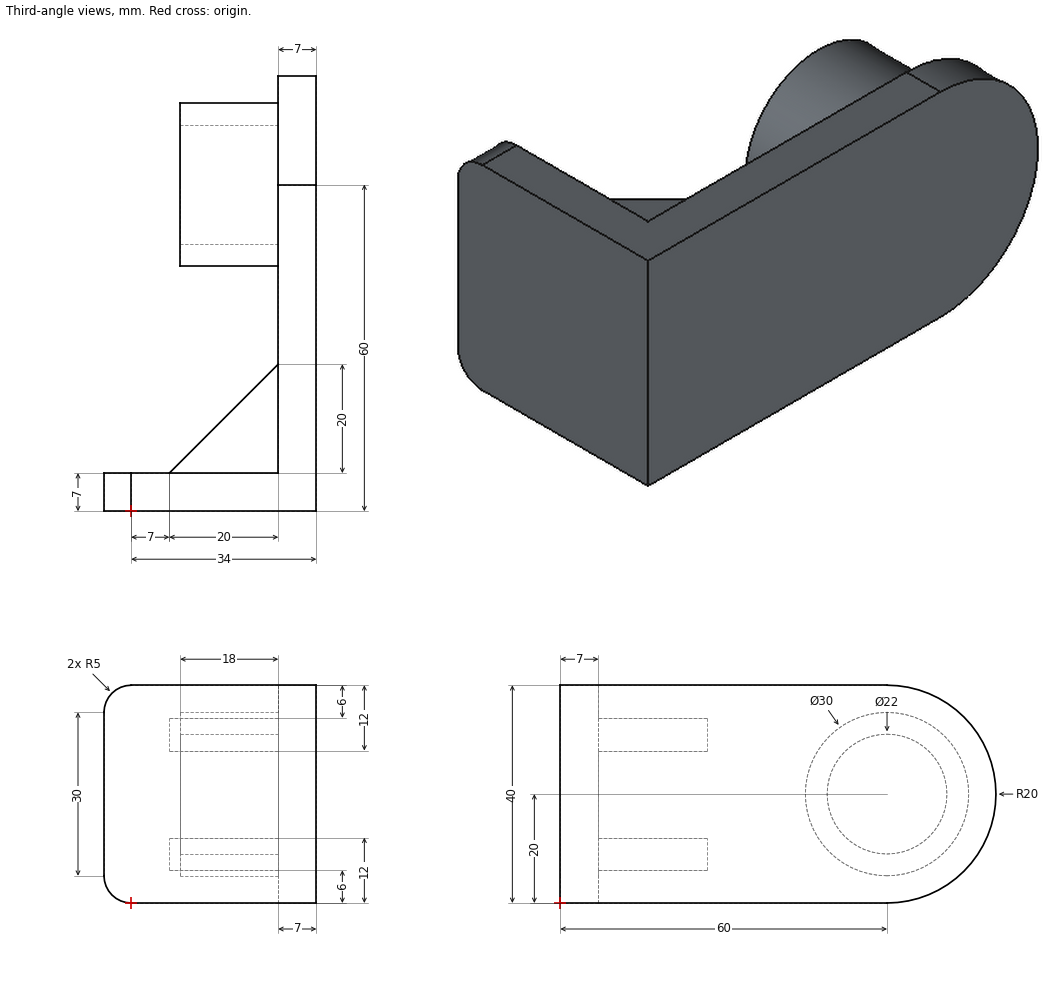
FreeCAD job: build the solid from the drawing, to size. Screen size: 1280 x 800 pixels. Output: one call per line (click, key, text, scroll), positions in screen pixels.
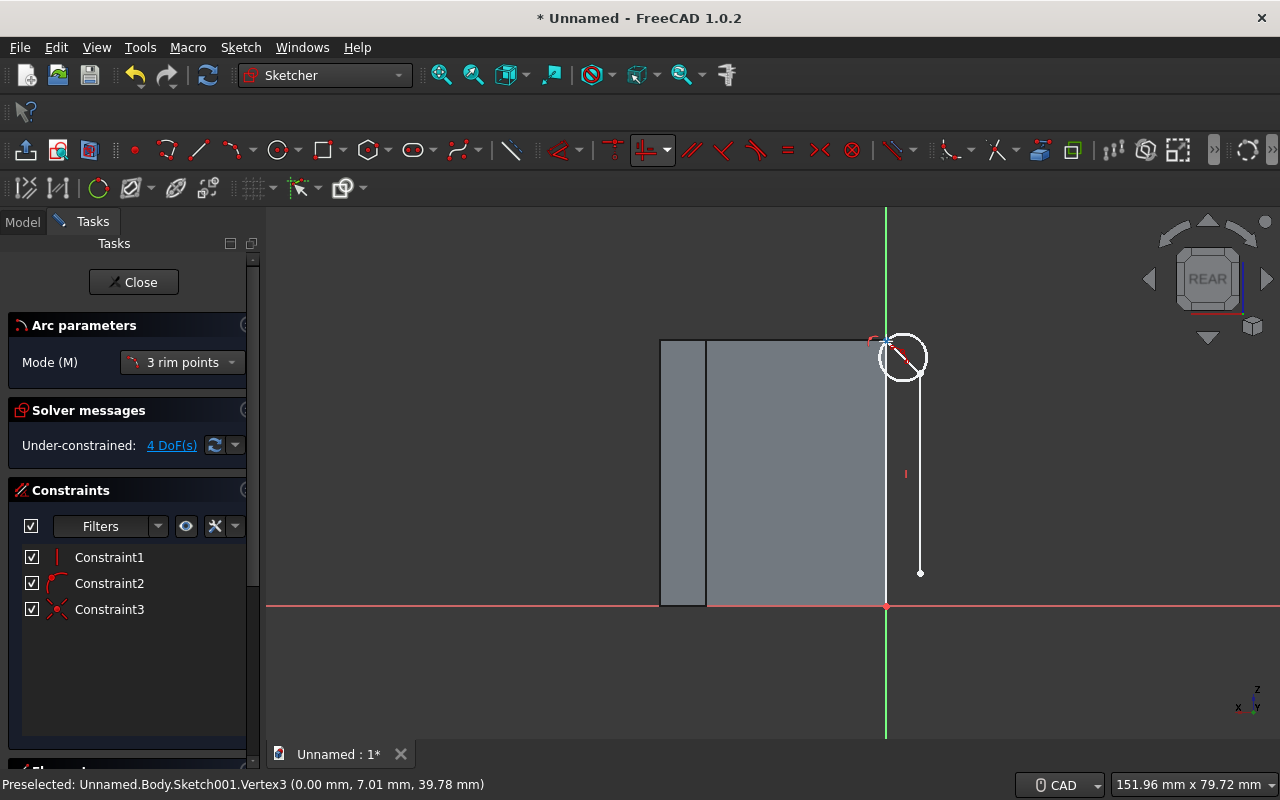
scroll(910, 349, up, 3)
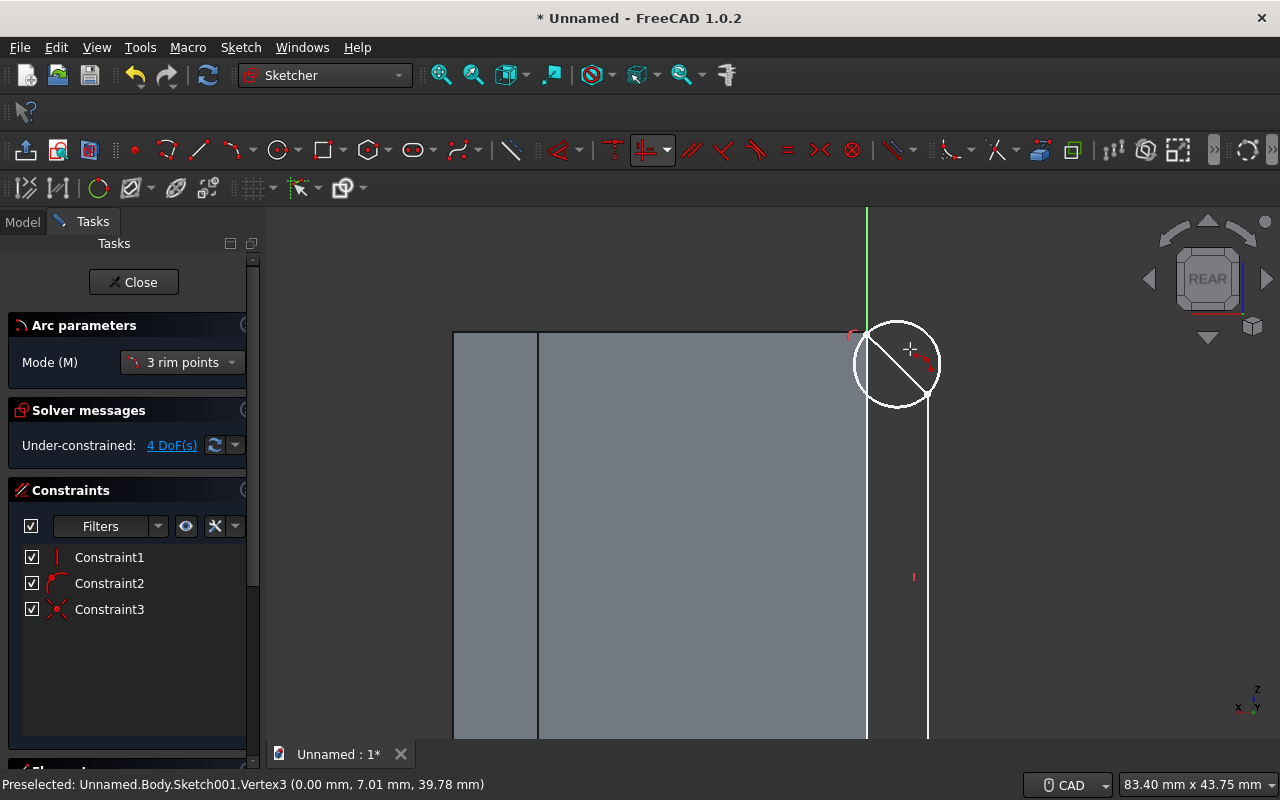
click(910, 349)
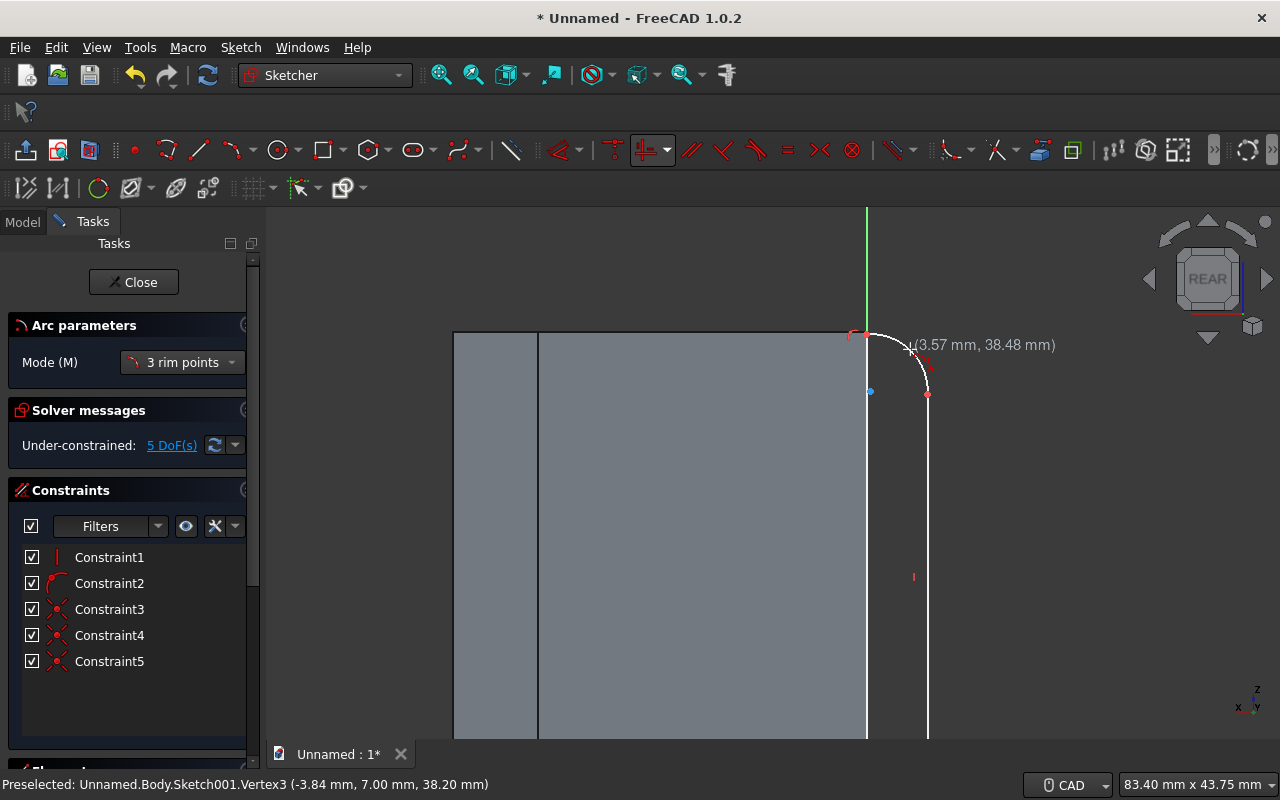
scroll(313, 266, down, 2)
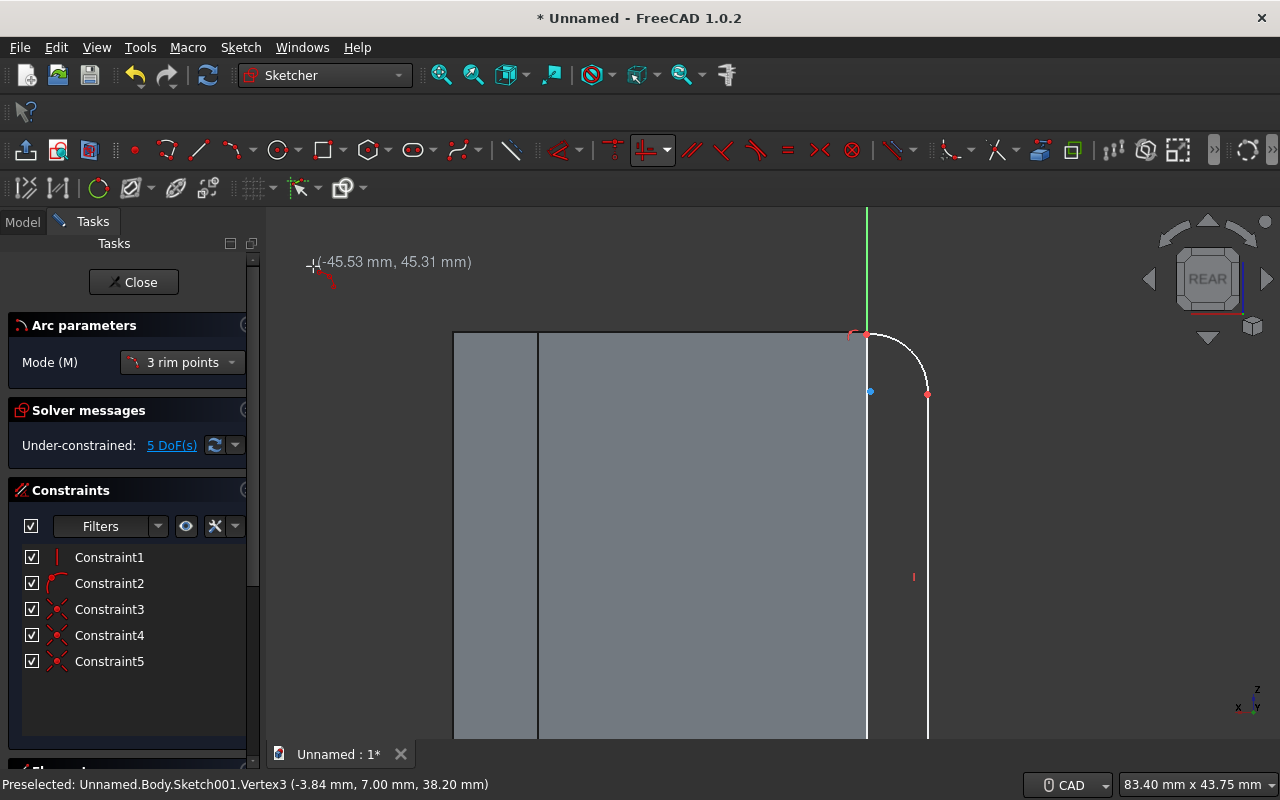
click(684, 636)
click(725, 596)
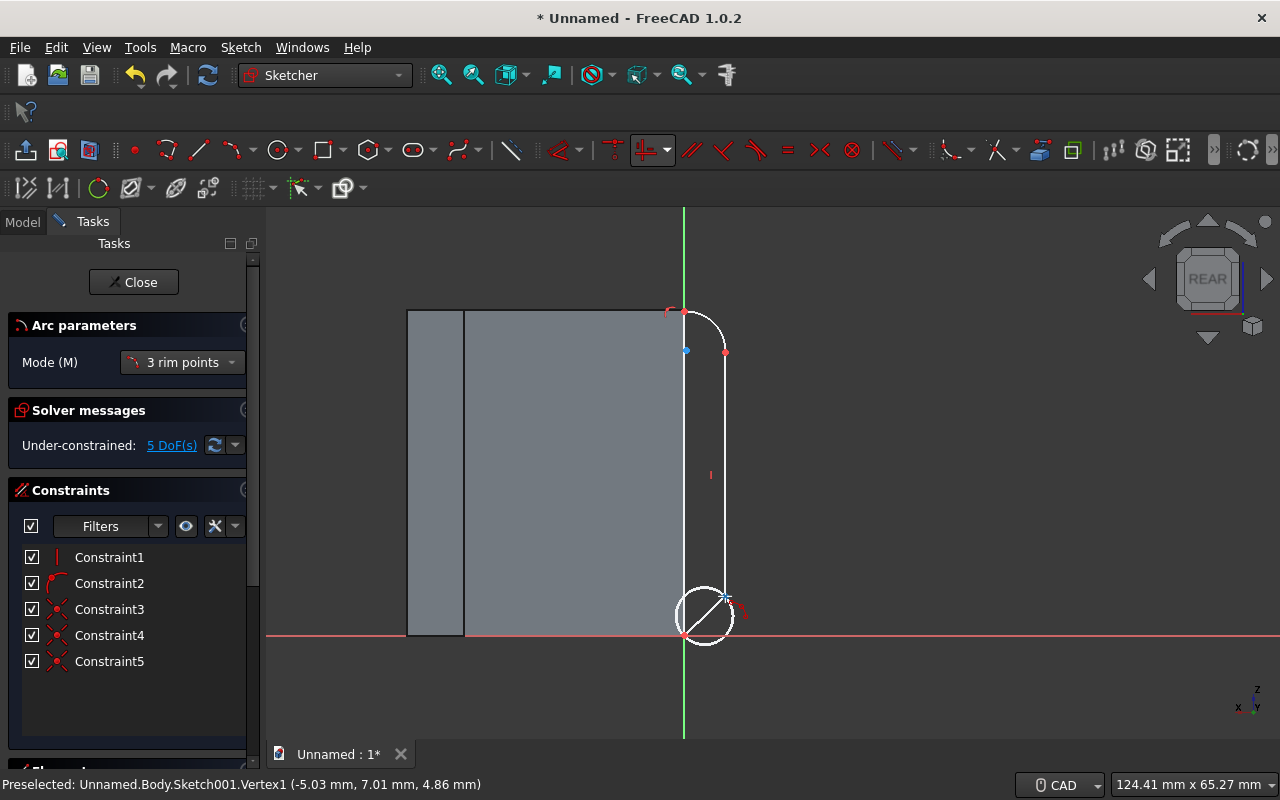
scroll(713, 624, up, 2)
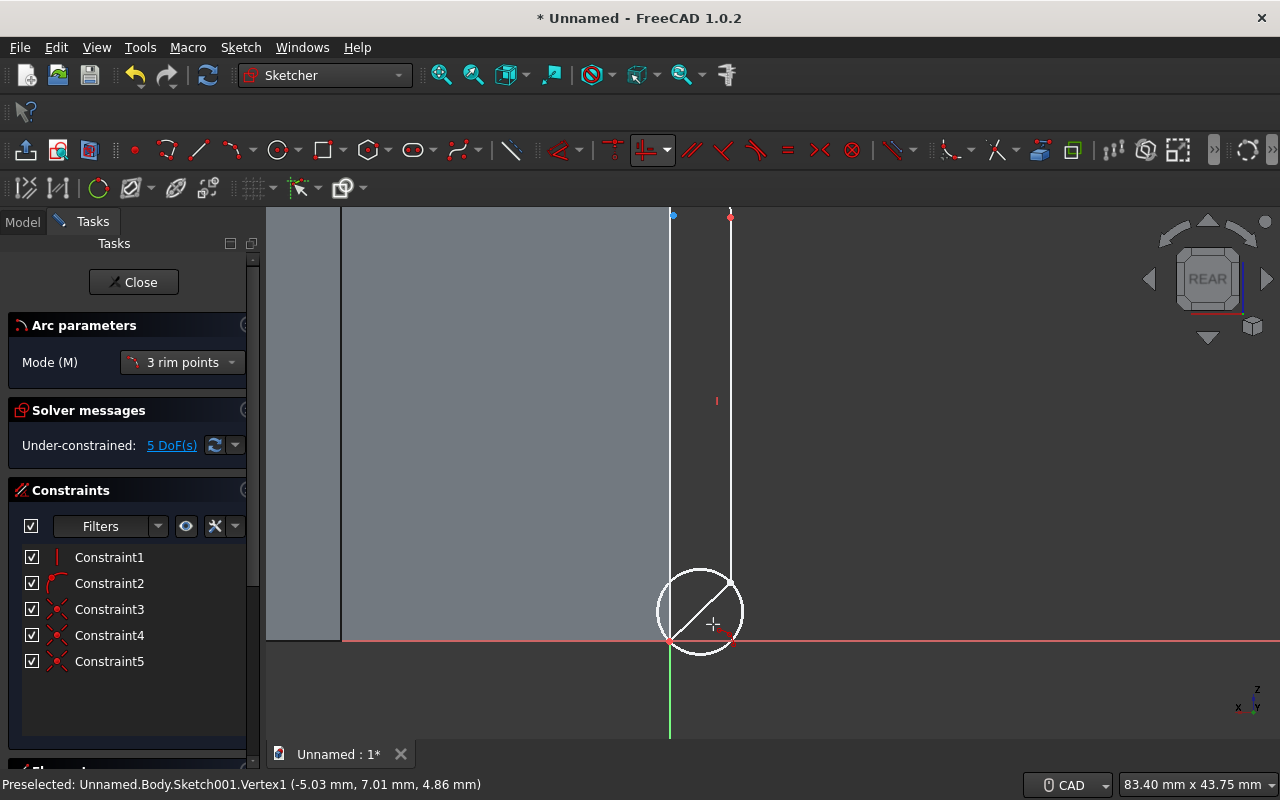
click(713, 624)
key(Escape)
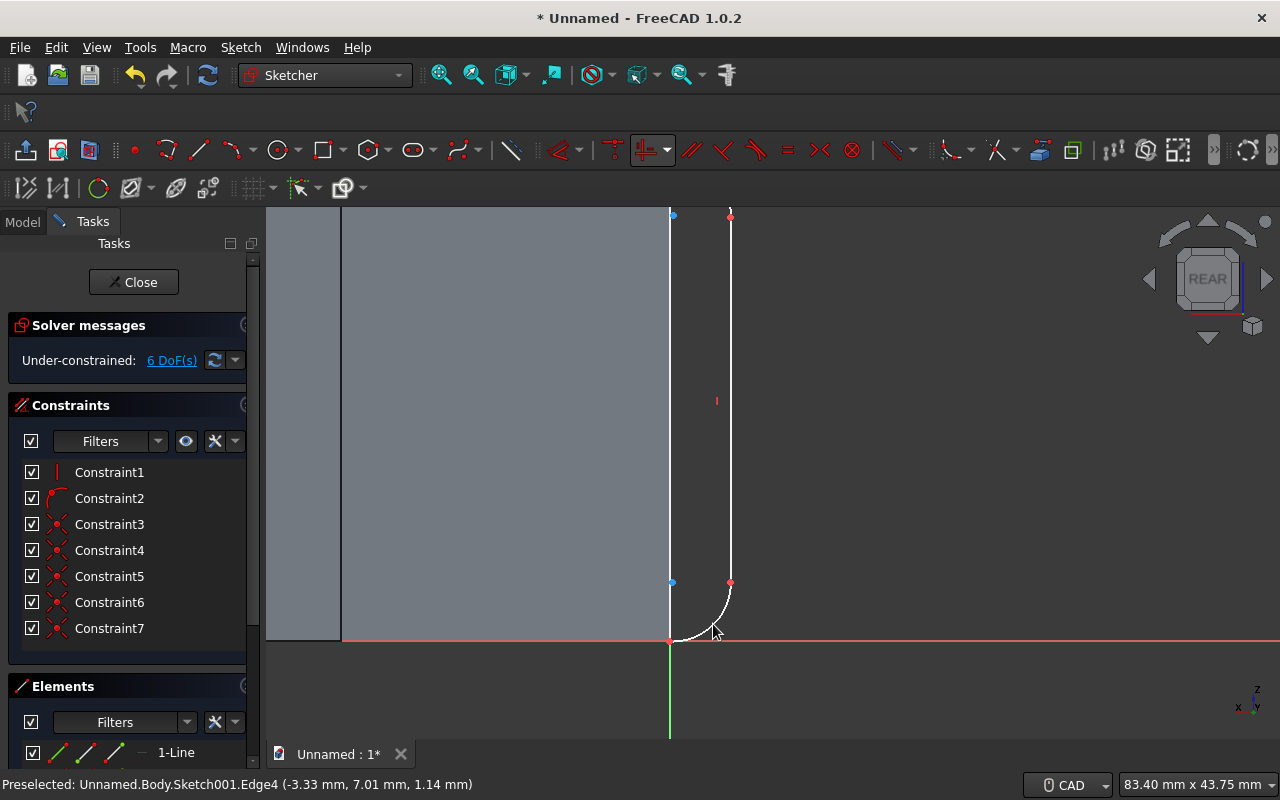
click(731, 473)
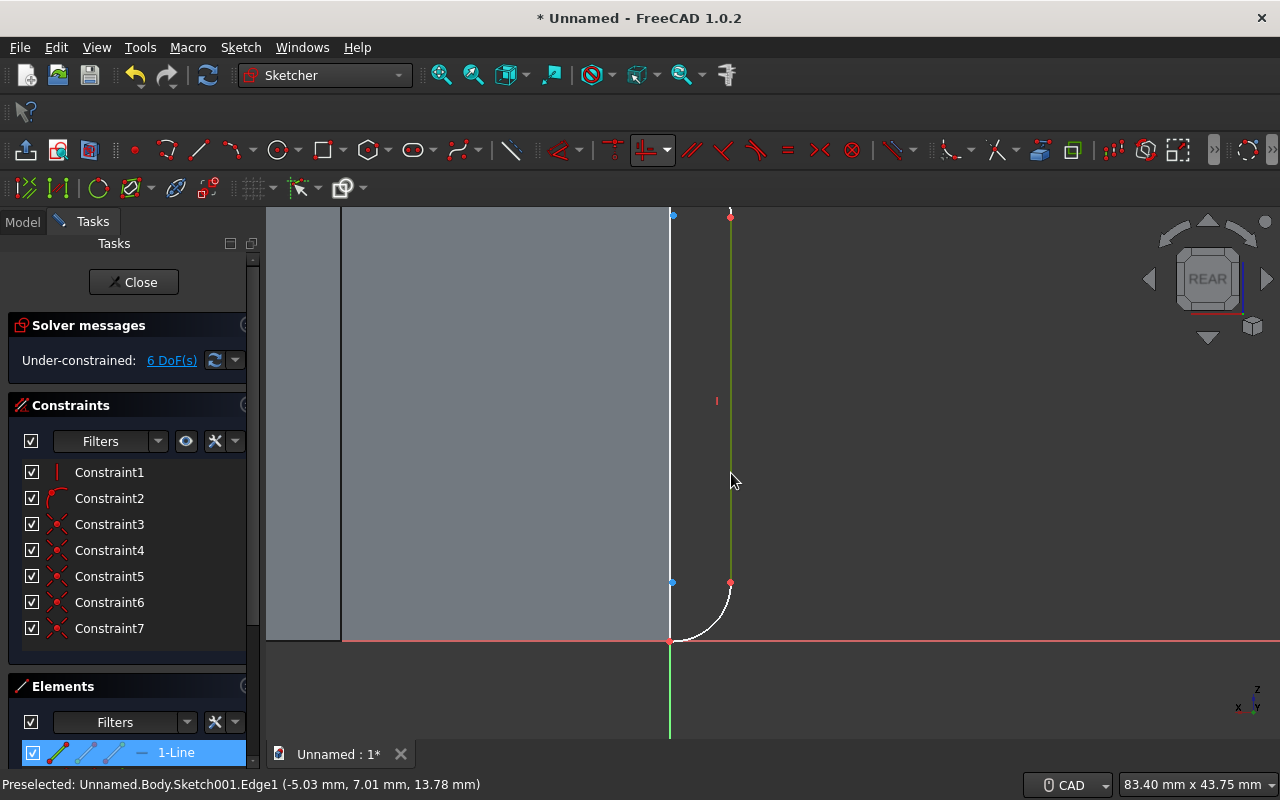
scroll(714, 625, down, 2)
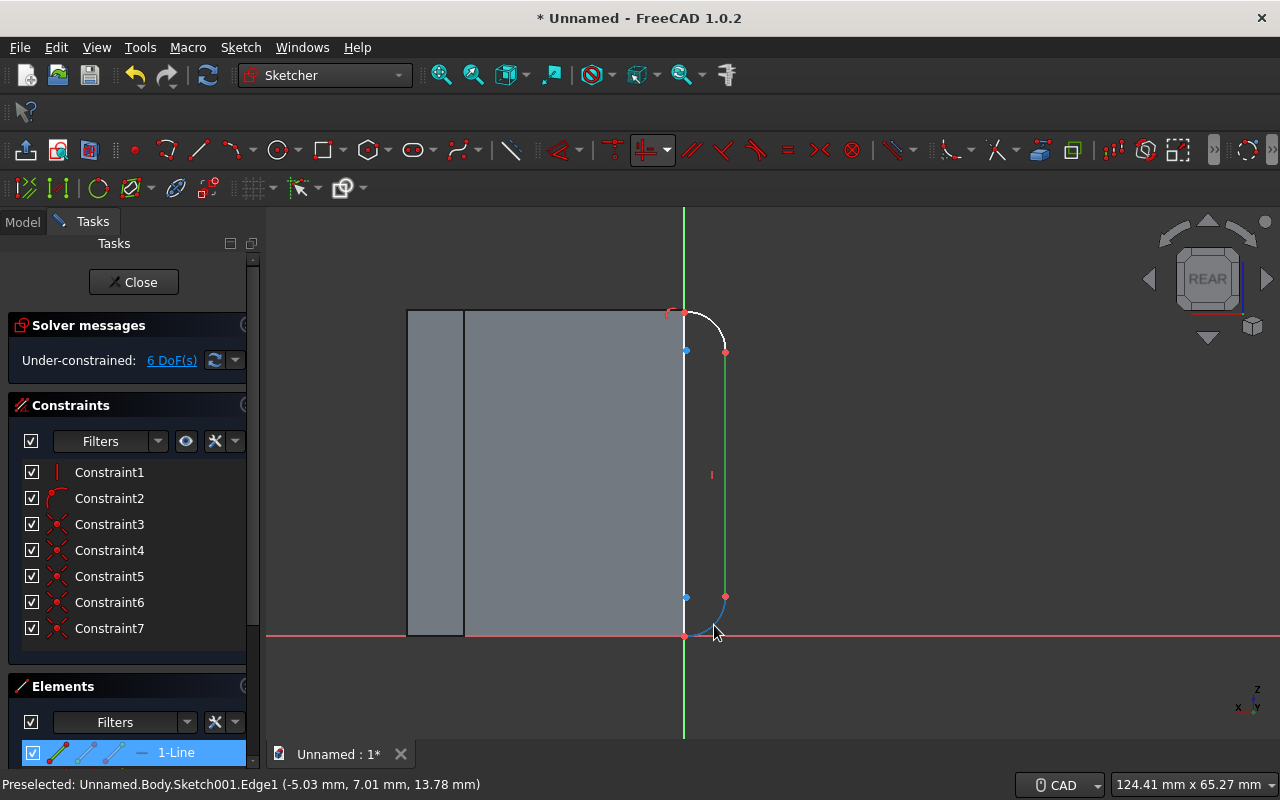
click(721, 334)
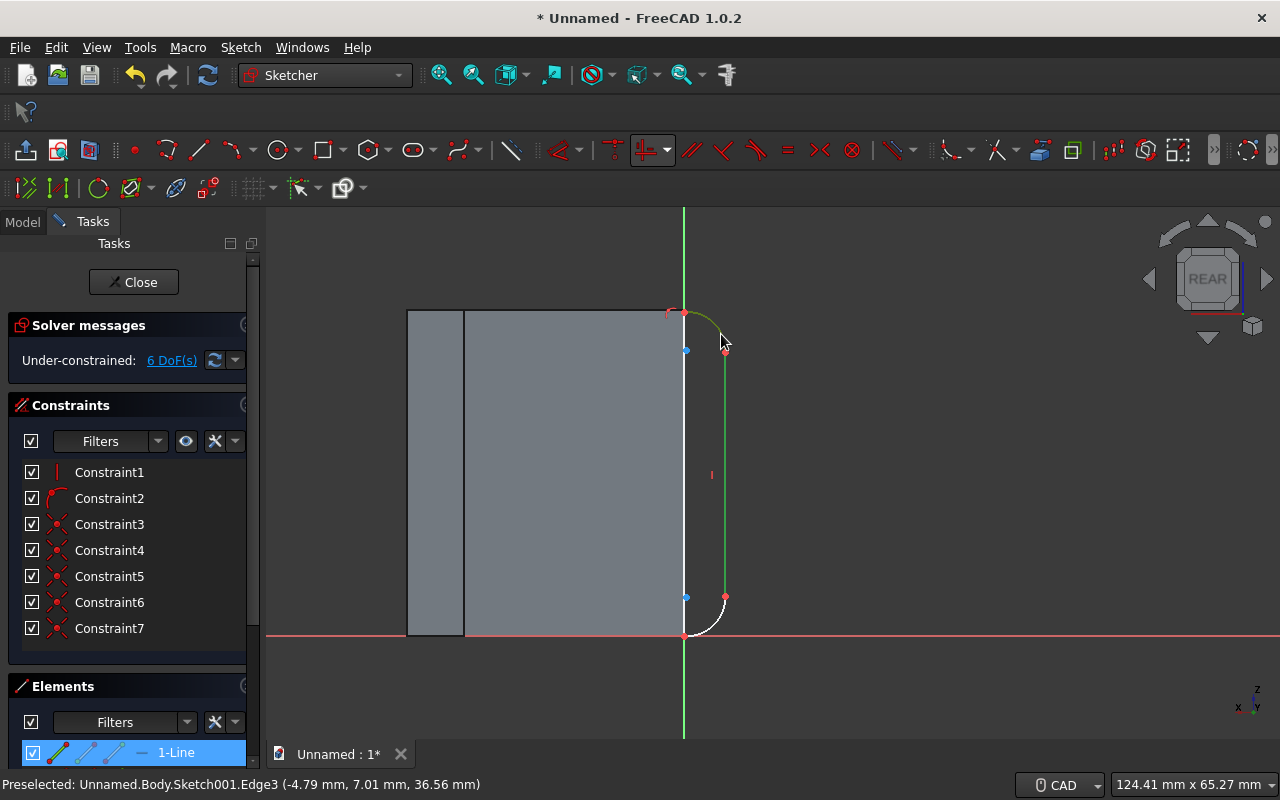
click(756, 150)